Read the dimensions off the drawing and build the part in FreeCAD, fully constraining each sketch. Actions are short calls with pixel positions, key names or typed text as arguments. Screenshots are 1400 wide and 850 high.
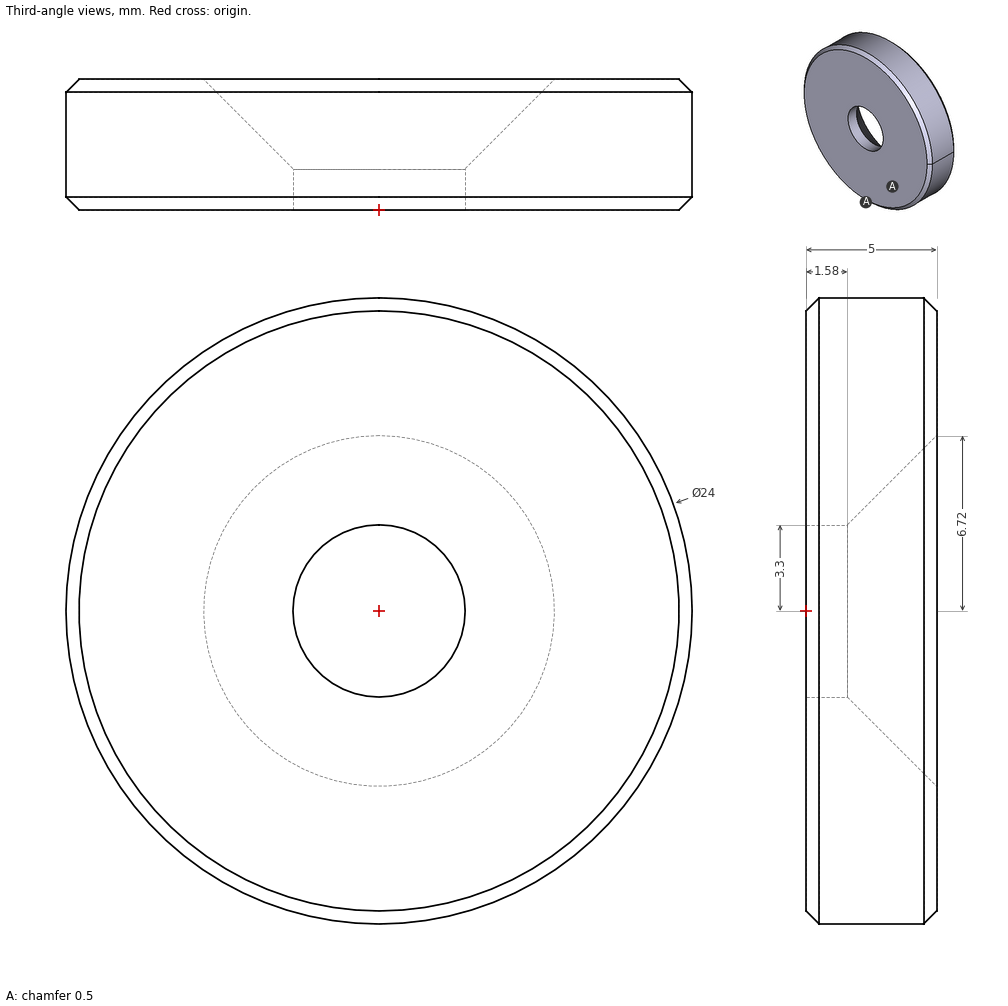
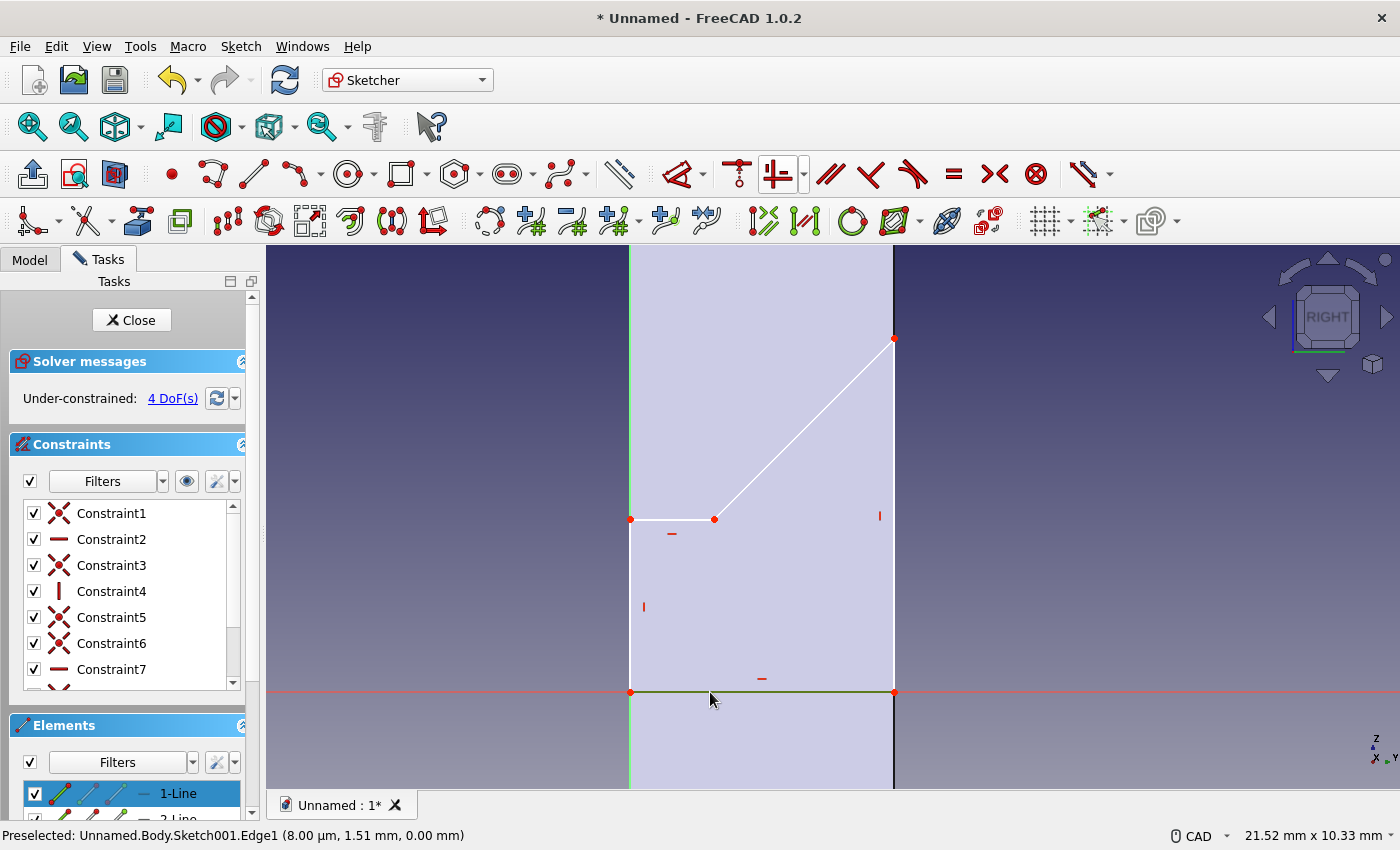
click(702, 174)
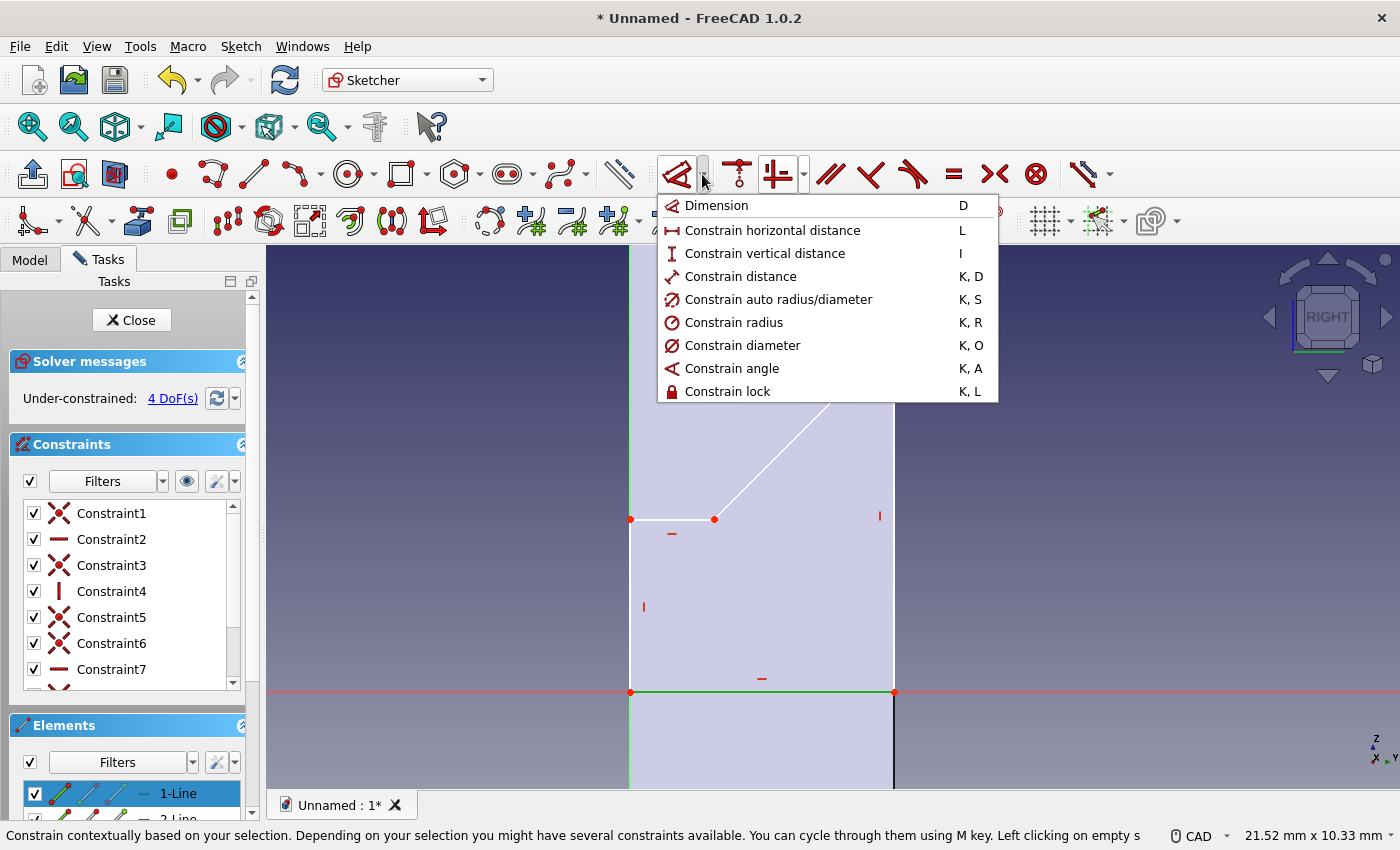
click(828, 230)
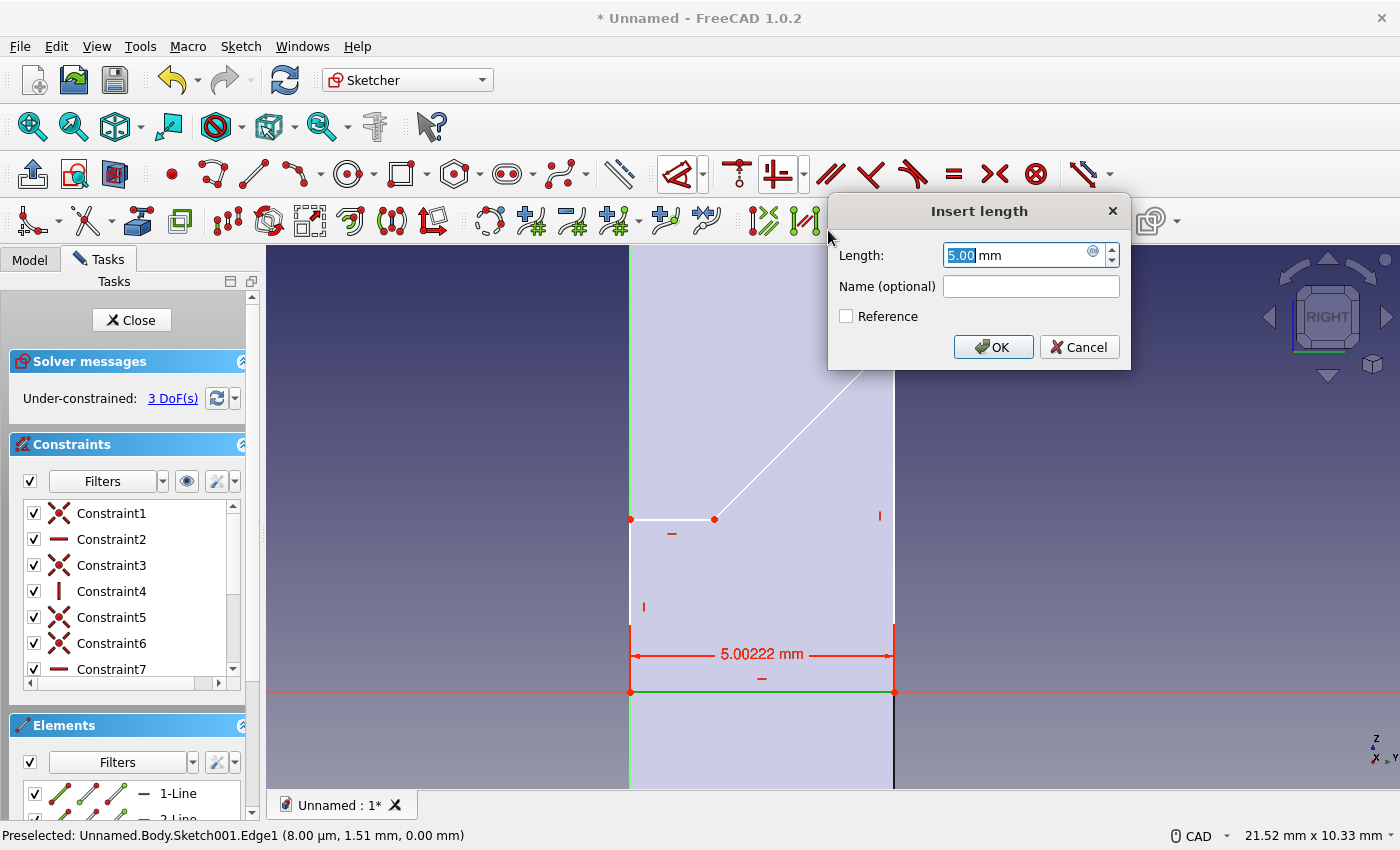
text(5)
key(Return)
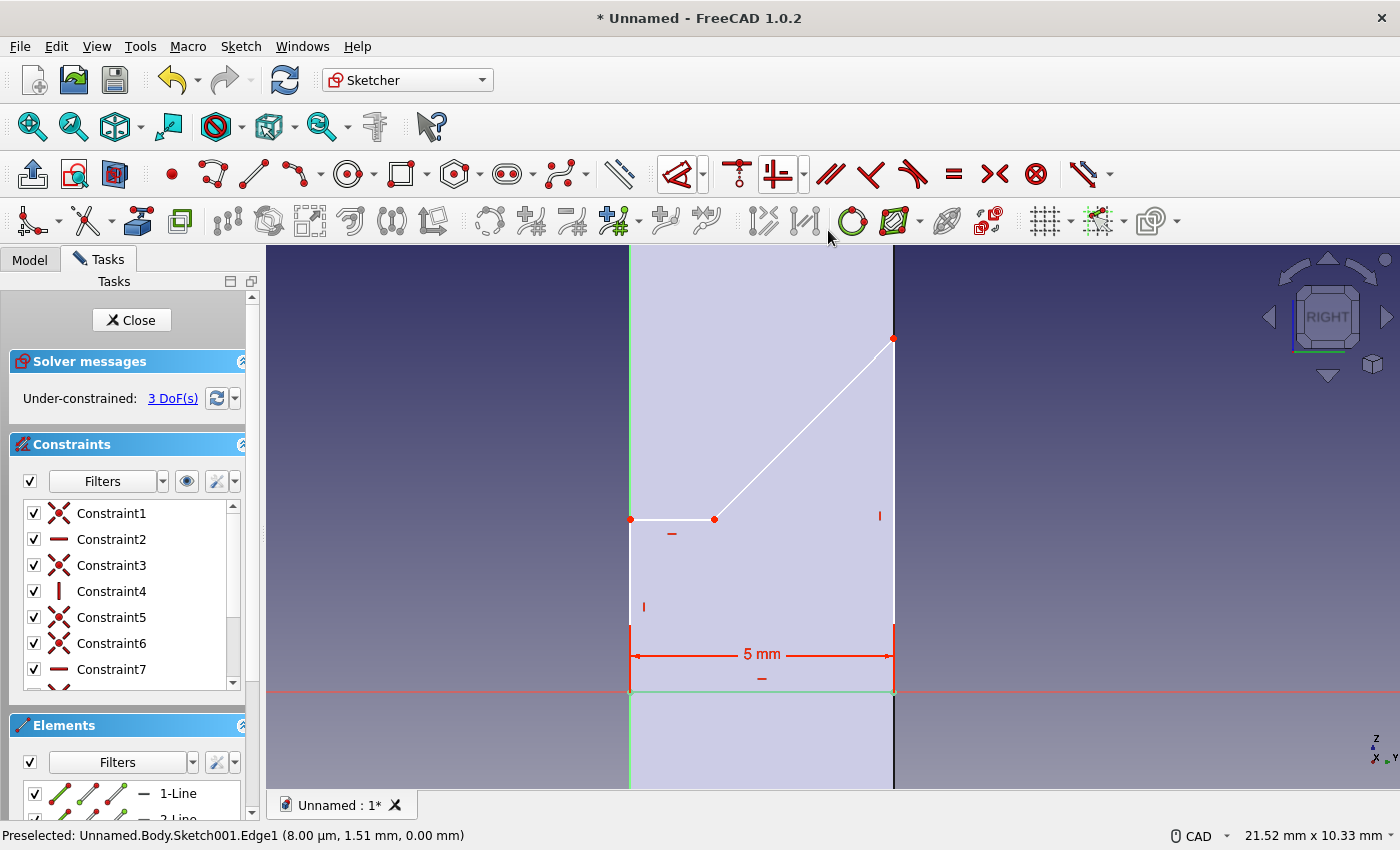
click(630, 572)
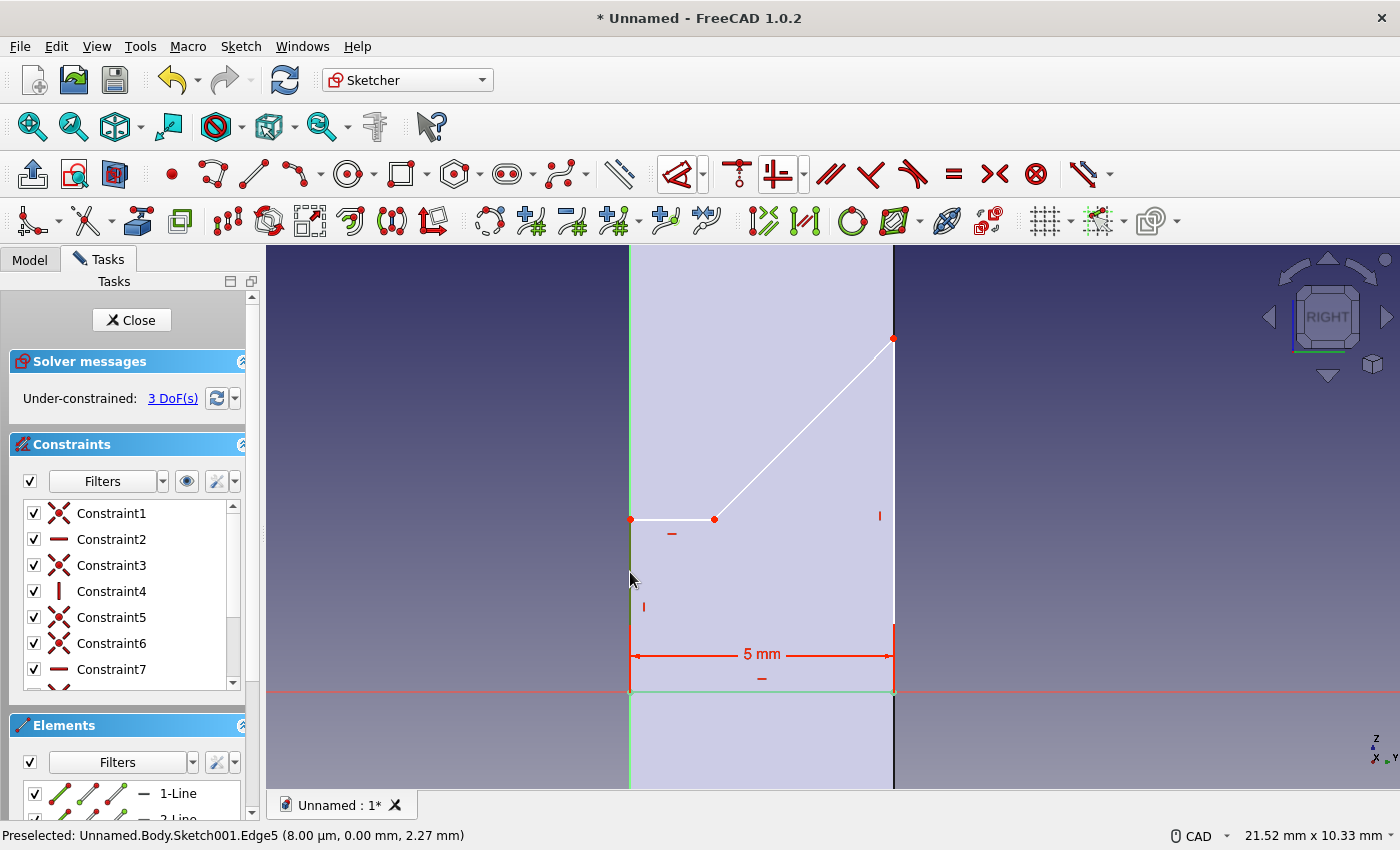
click(702, 174)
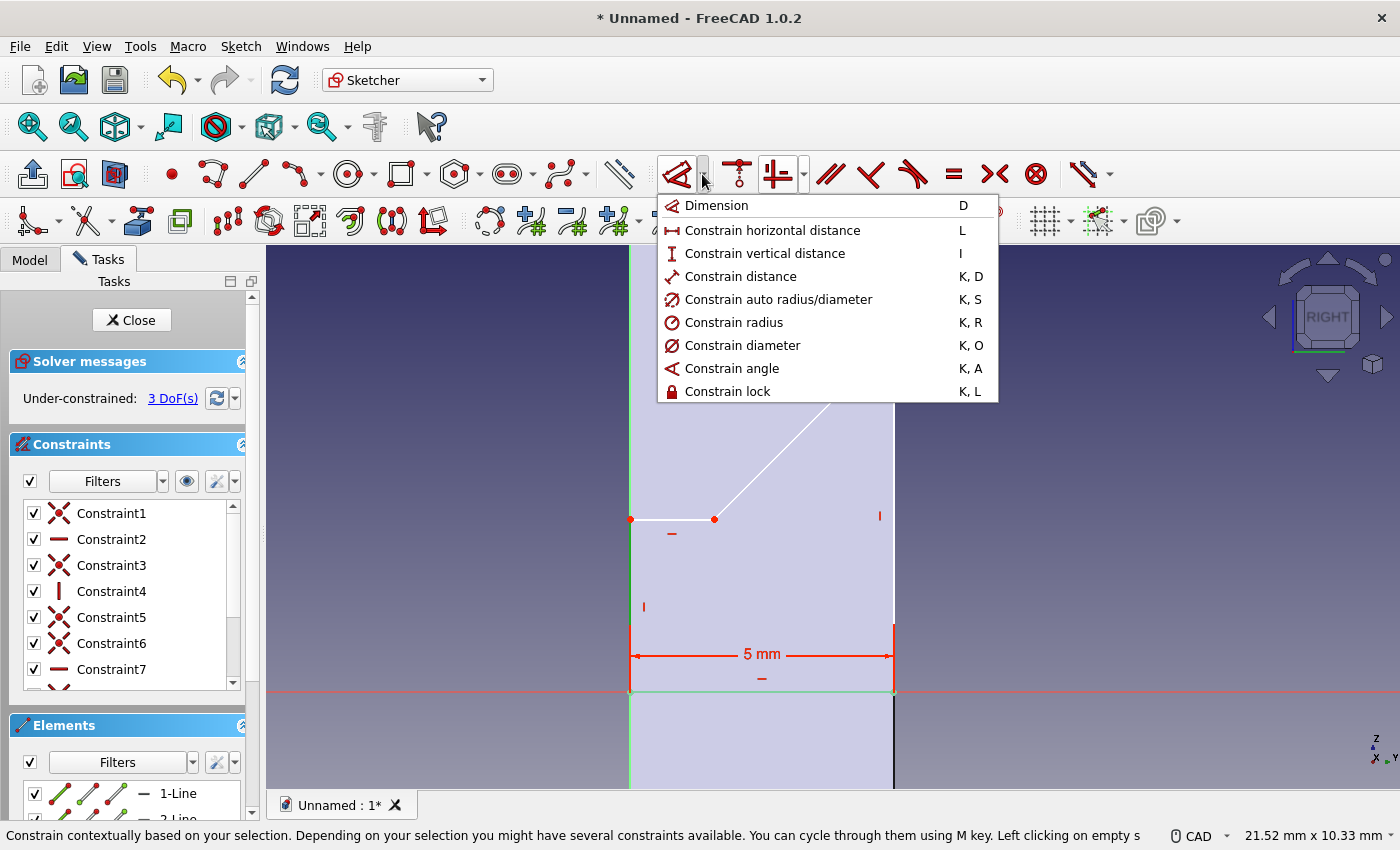
click(828, 254)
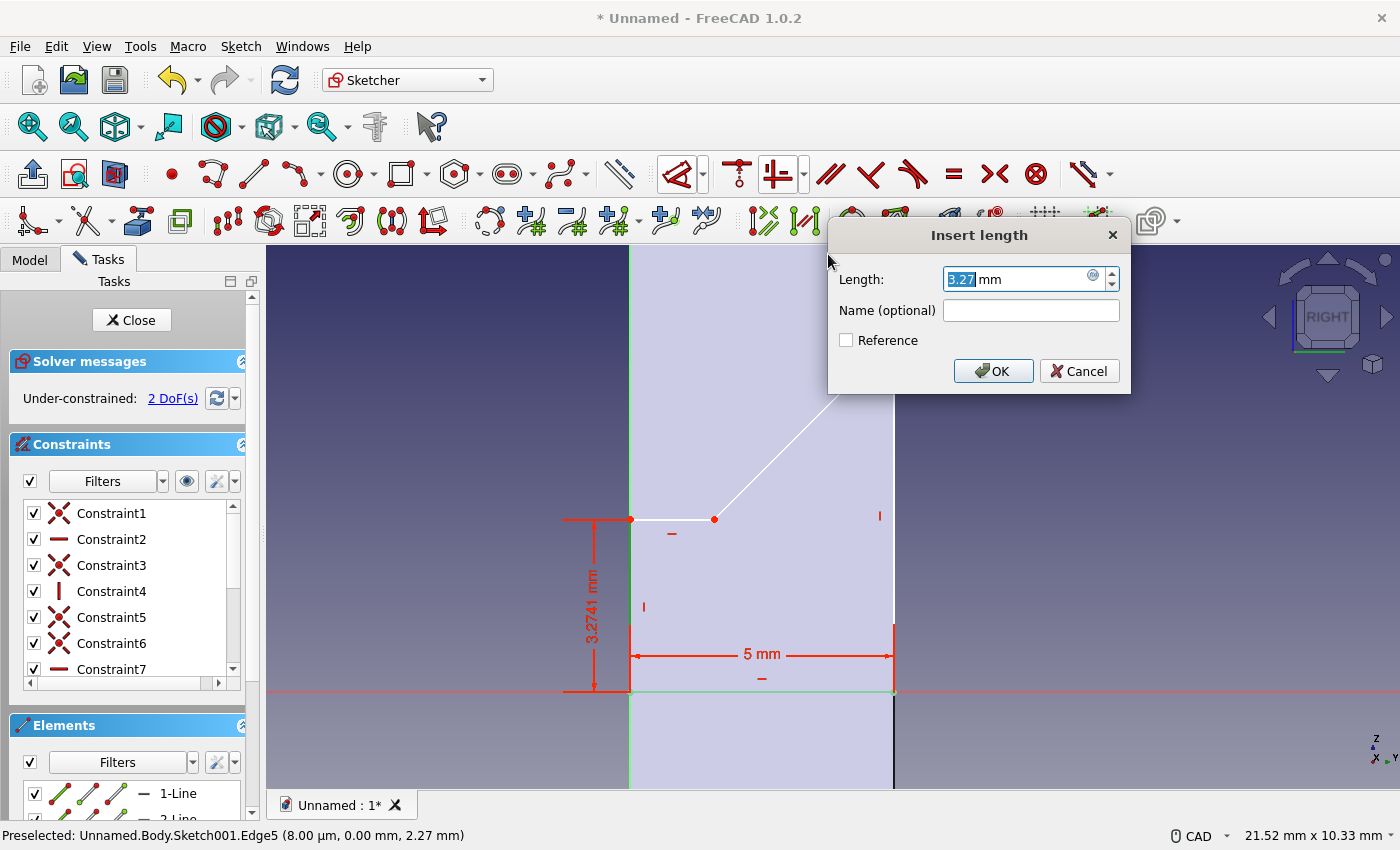
text(3.3)
key(Return)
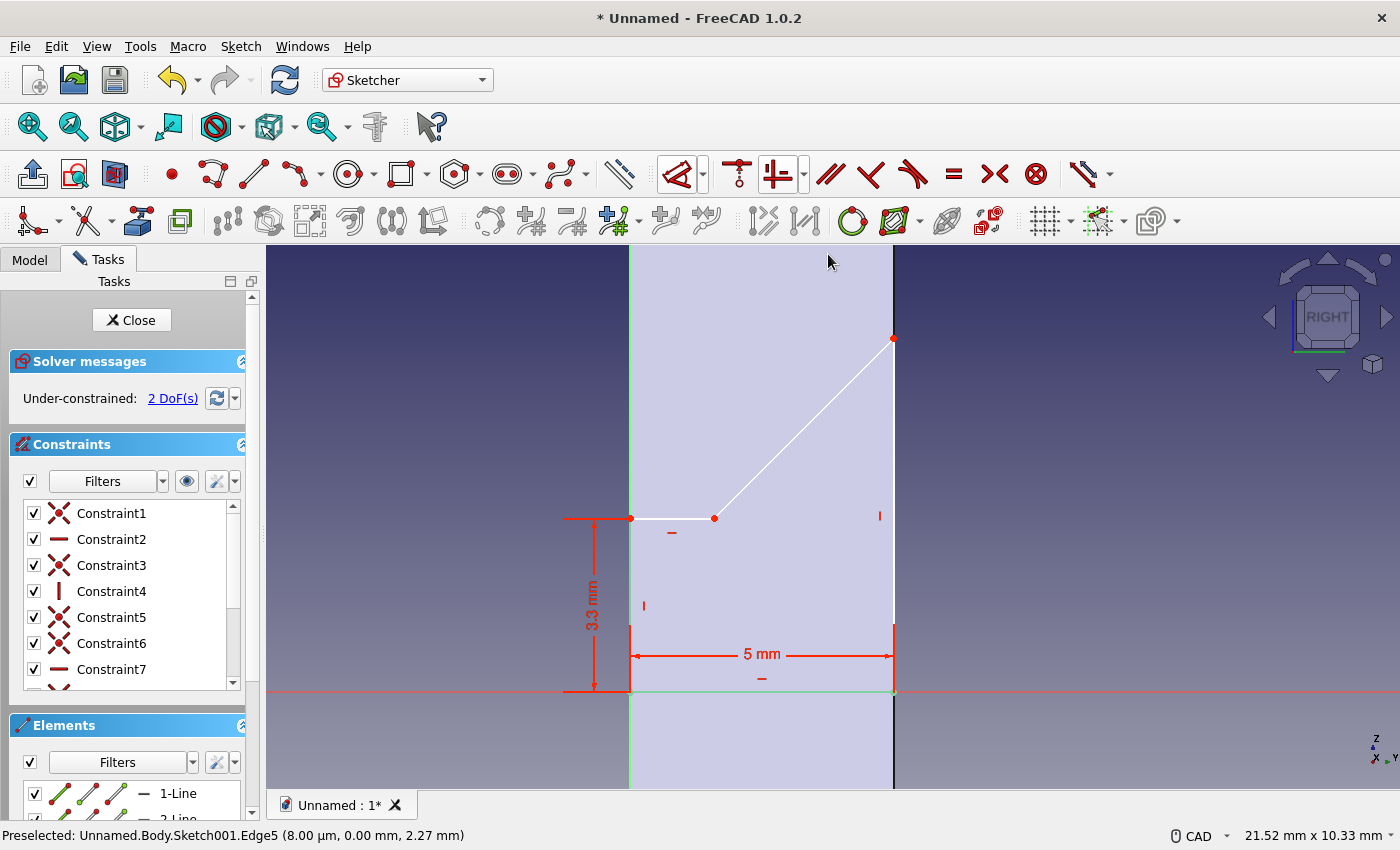
click(894, 586)